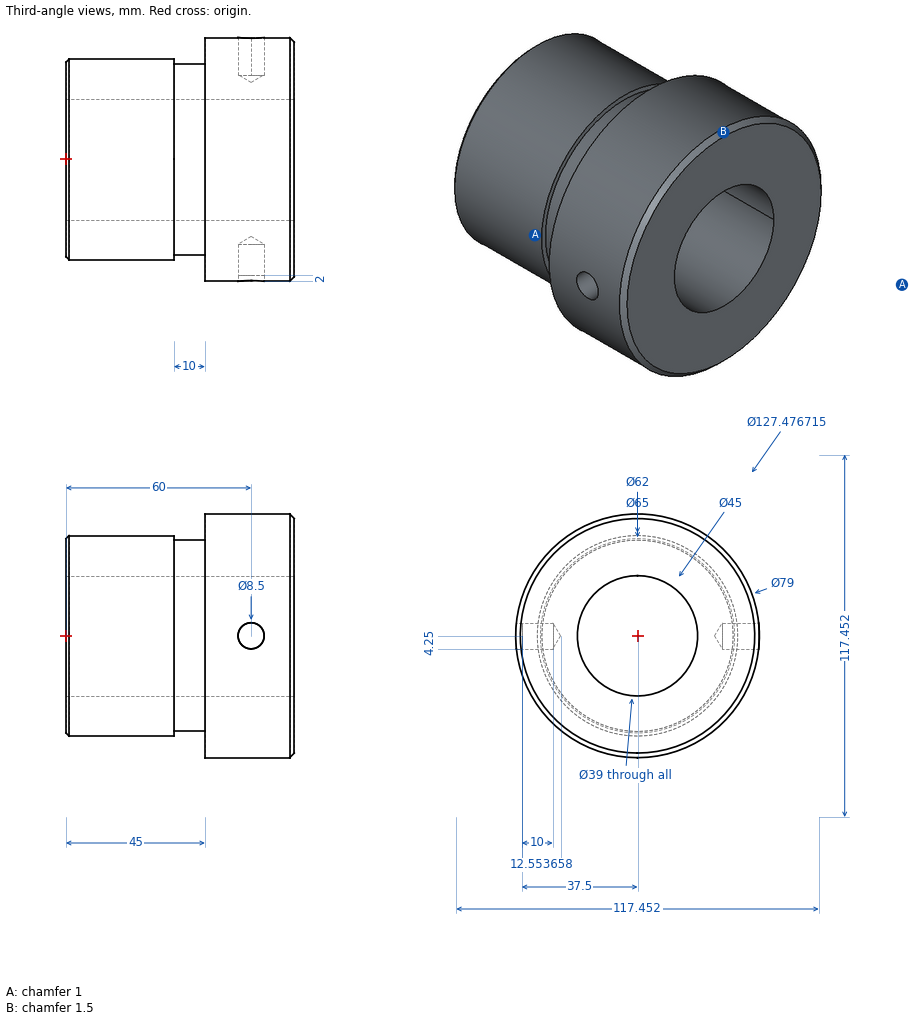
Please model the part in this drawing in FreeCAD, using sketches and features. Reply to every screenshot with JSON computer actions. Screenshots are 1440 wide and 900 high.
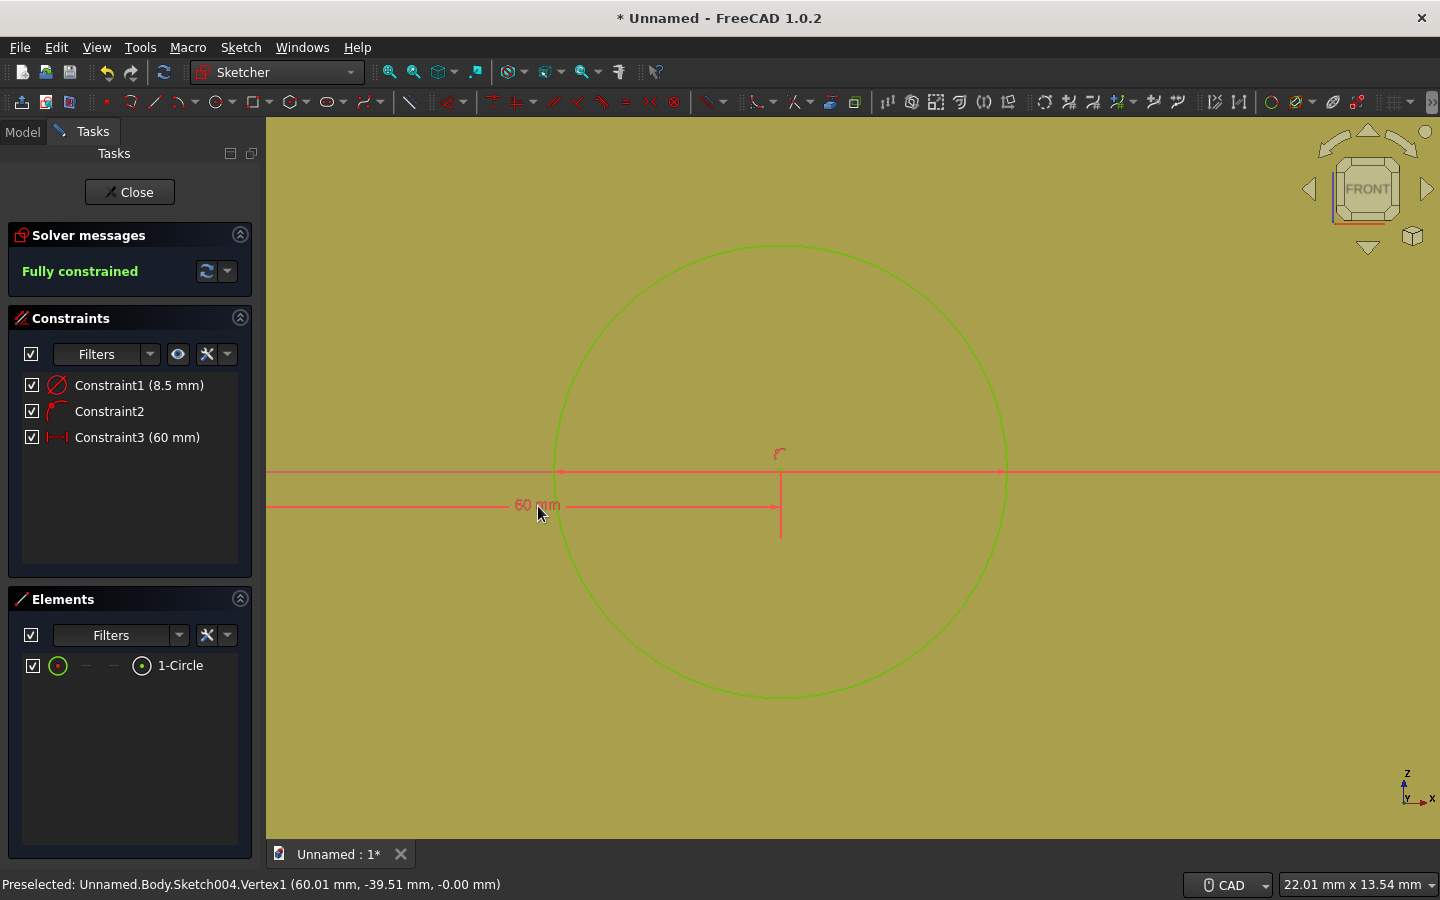
{"action": "left_click", "coordinate": [130, 192]}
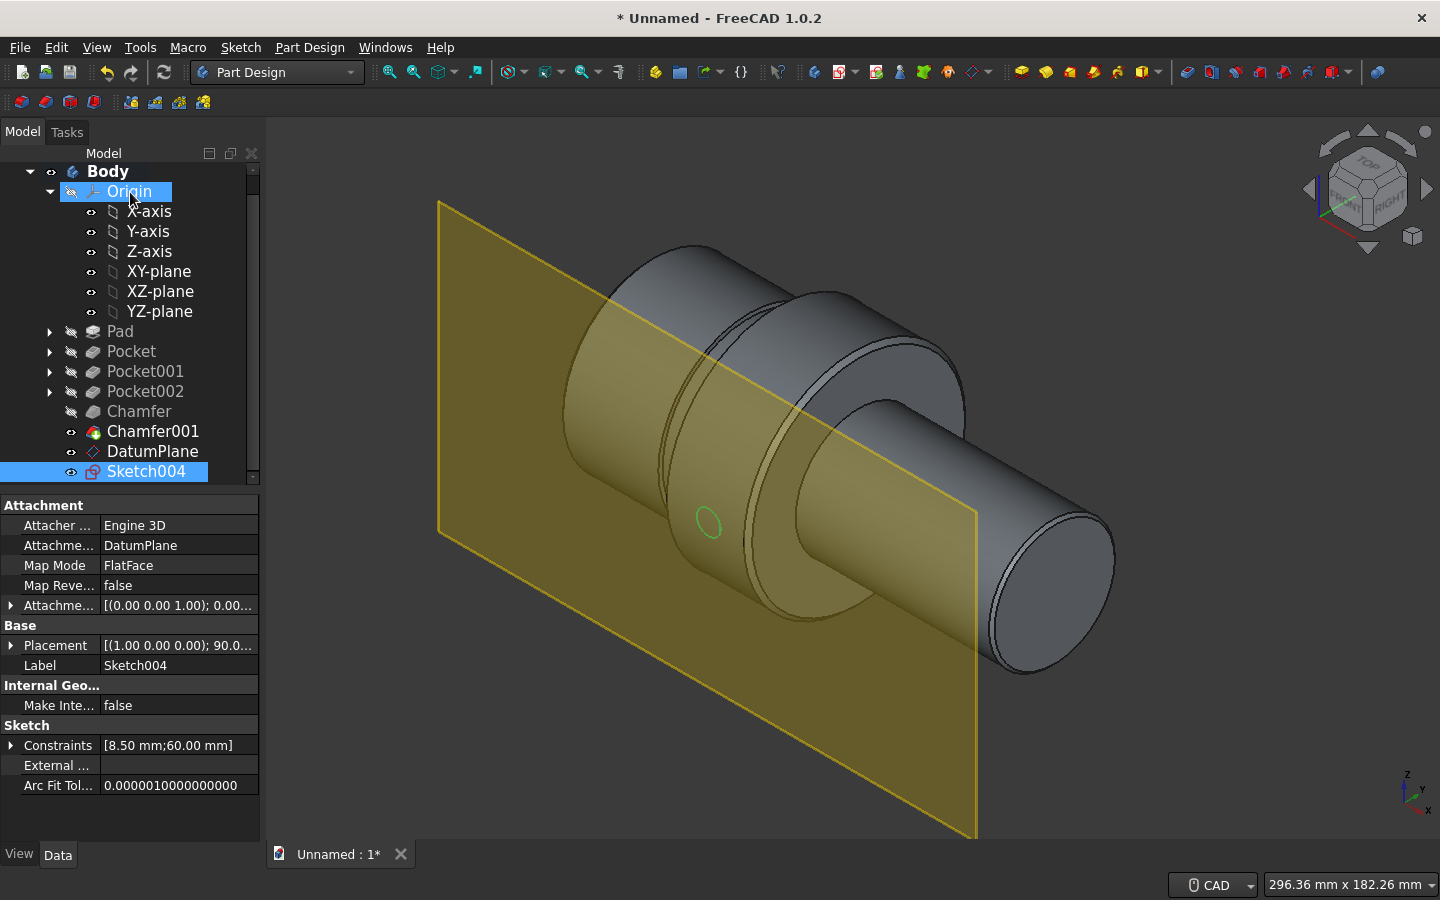
{"action": "left_click", "coordinate": [1188, 72]}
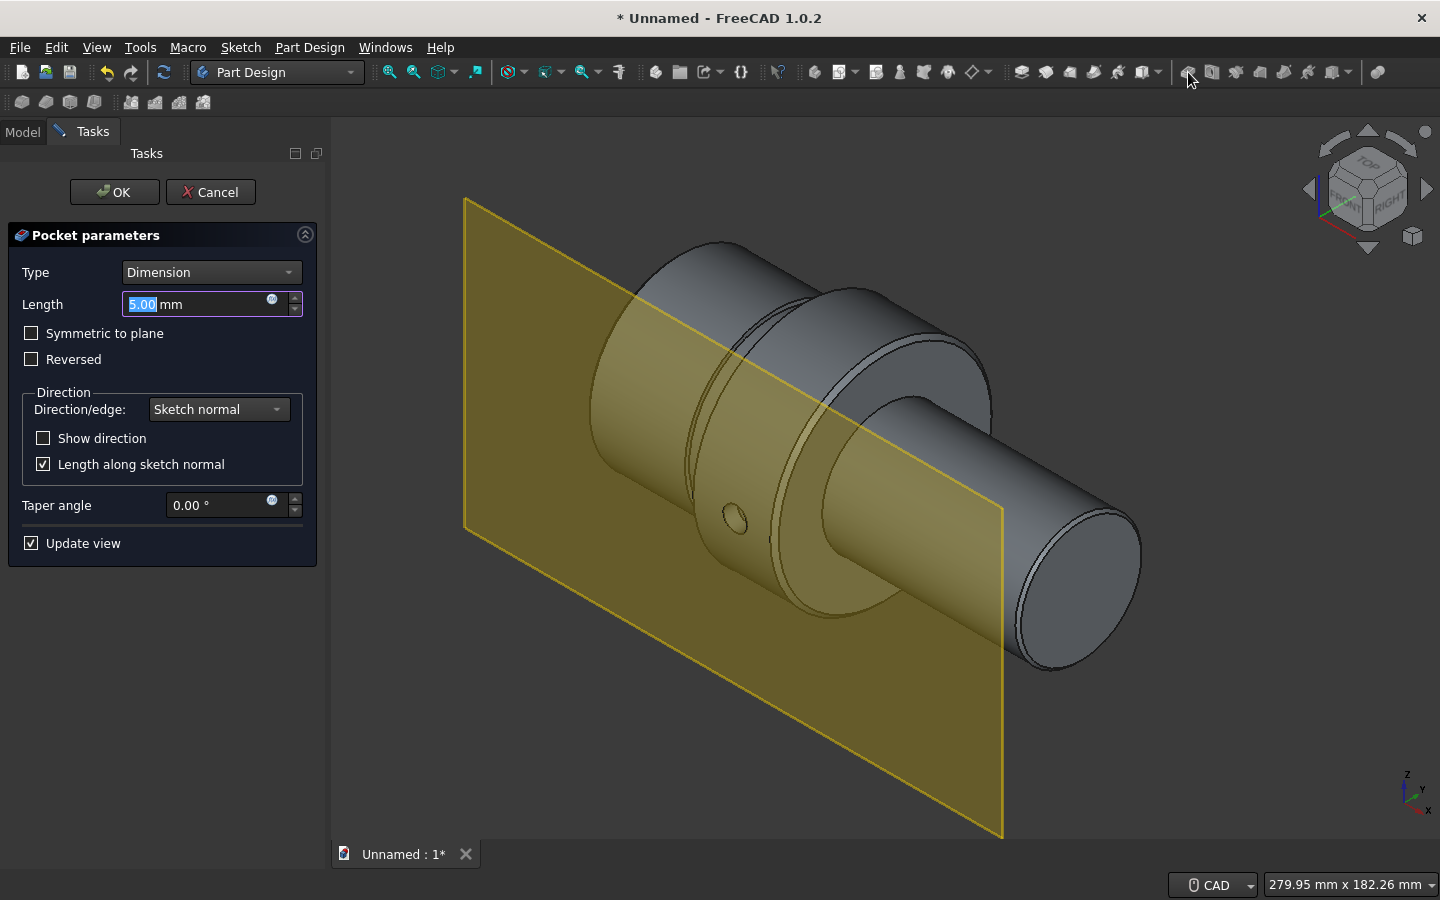
{"action": "type", "text": "2"}
{"action": "key", "text": "Tab"}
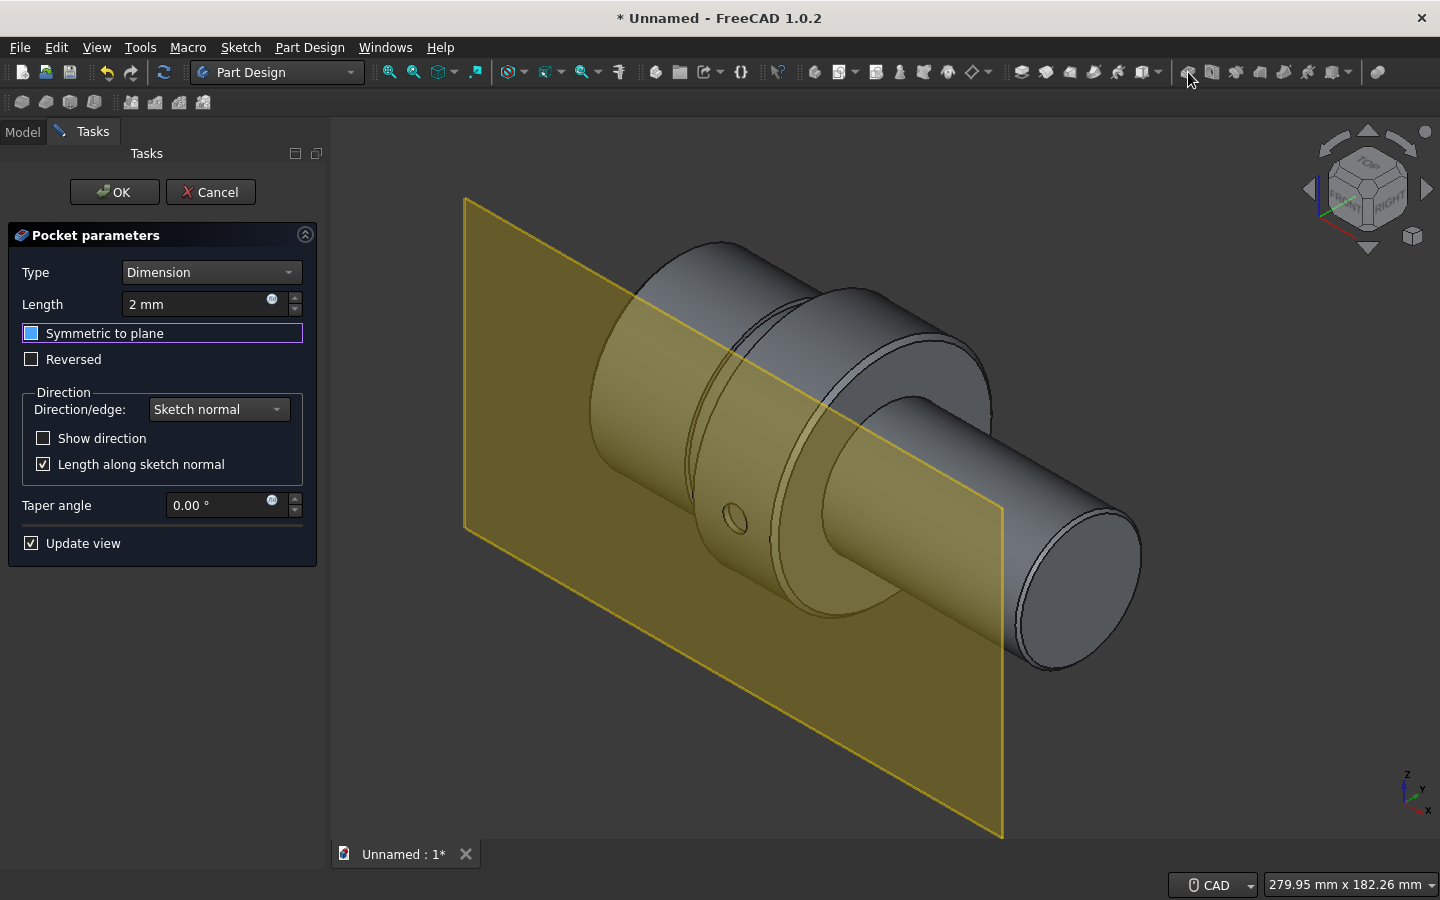
{"action": "left_click", "coordinate": [115, 192]}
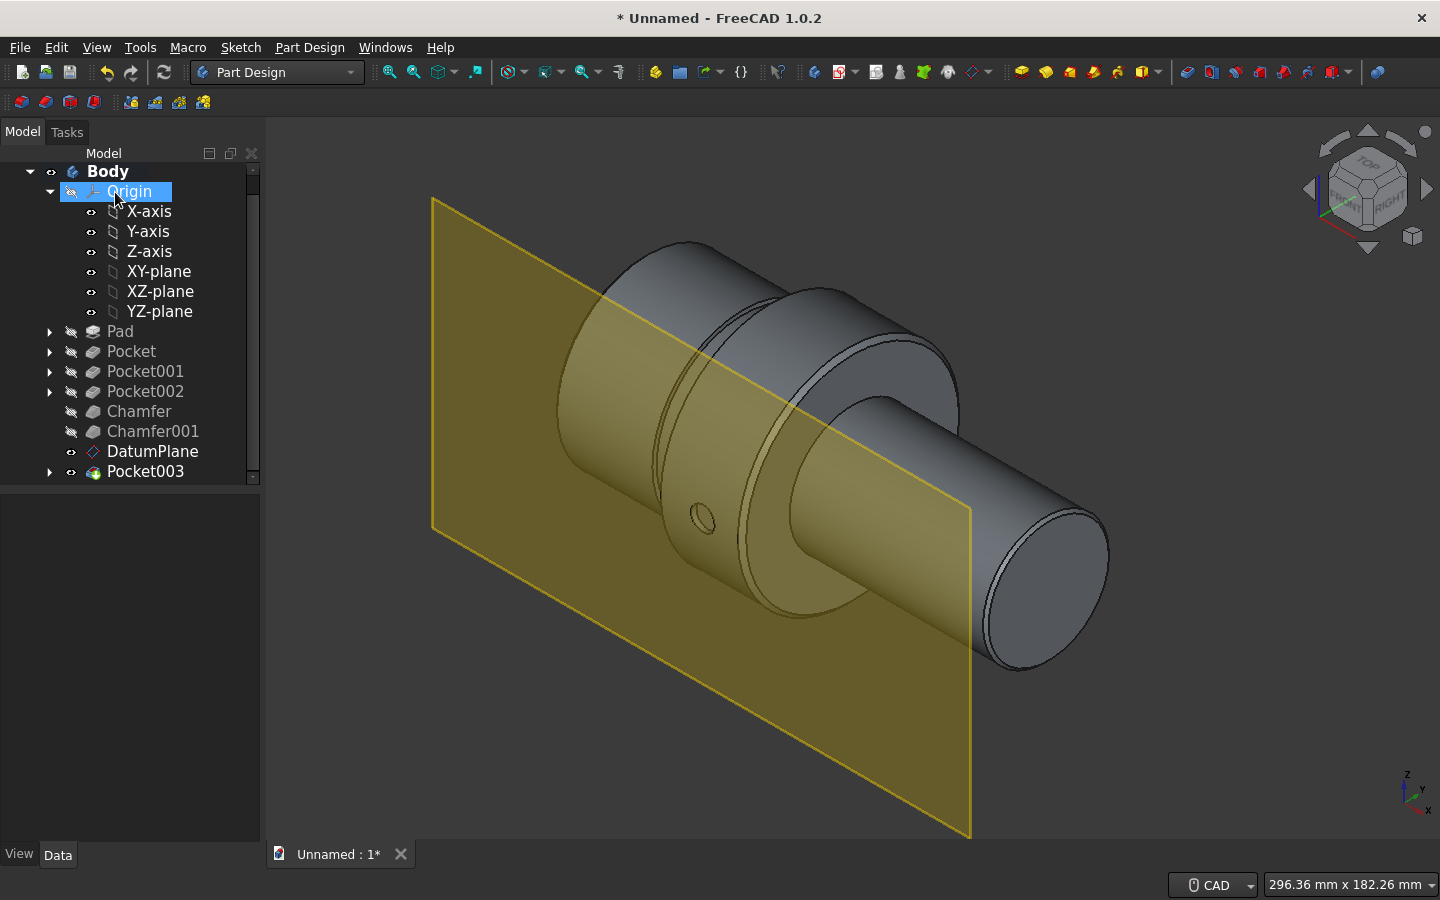
{"action": "left_click", "coordinate": [116, 452]}
{"action": "key", "text": "space"}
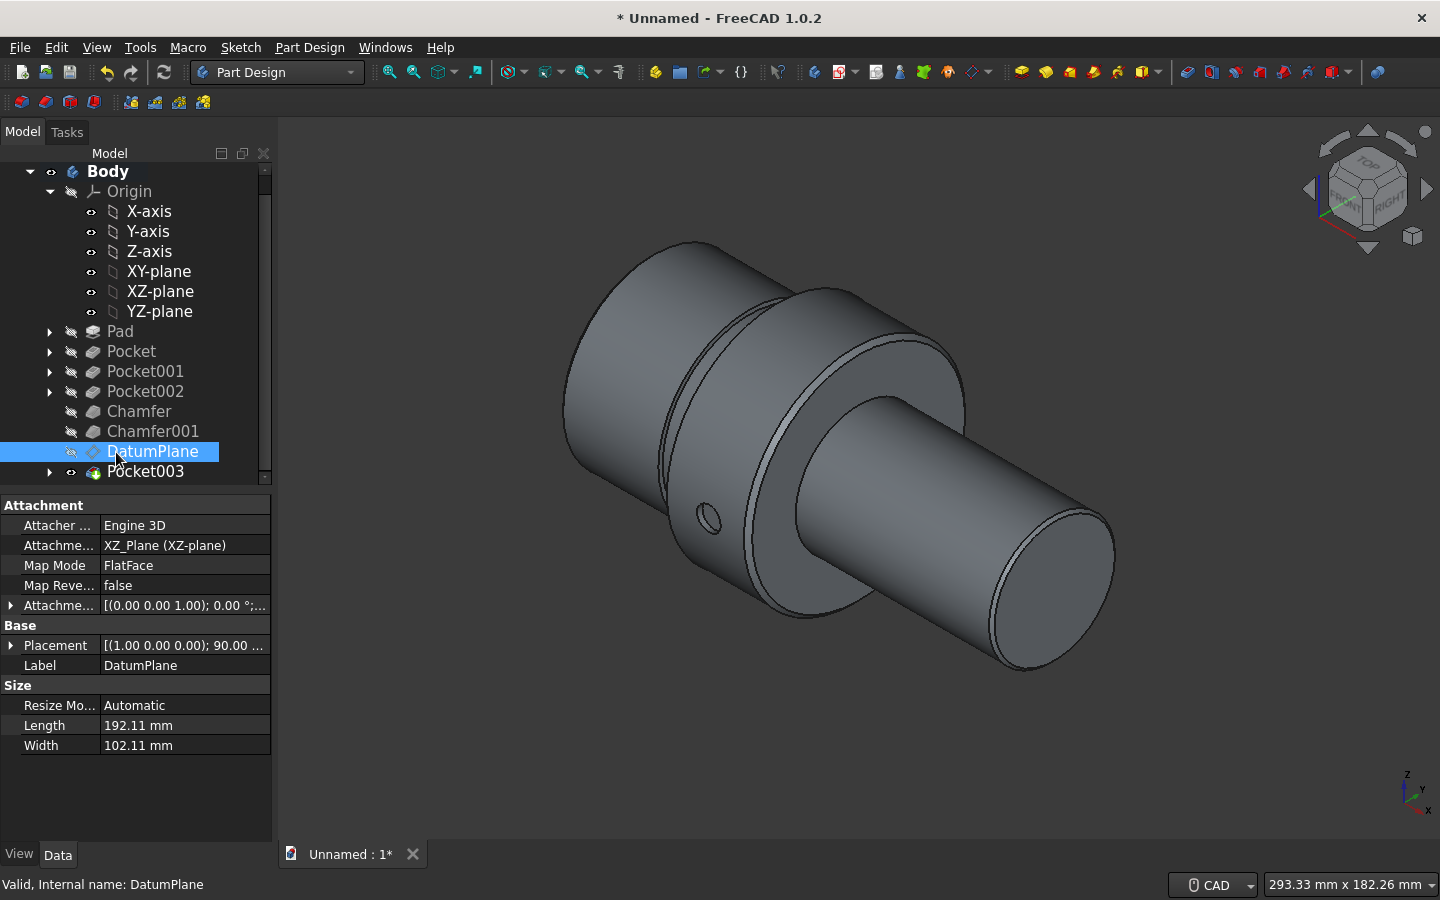
{"action": "left_click", "coordinate": [136, 312]}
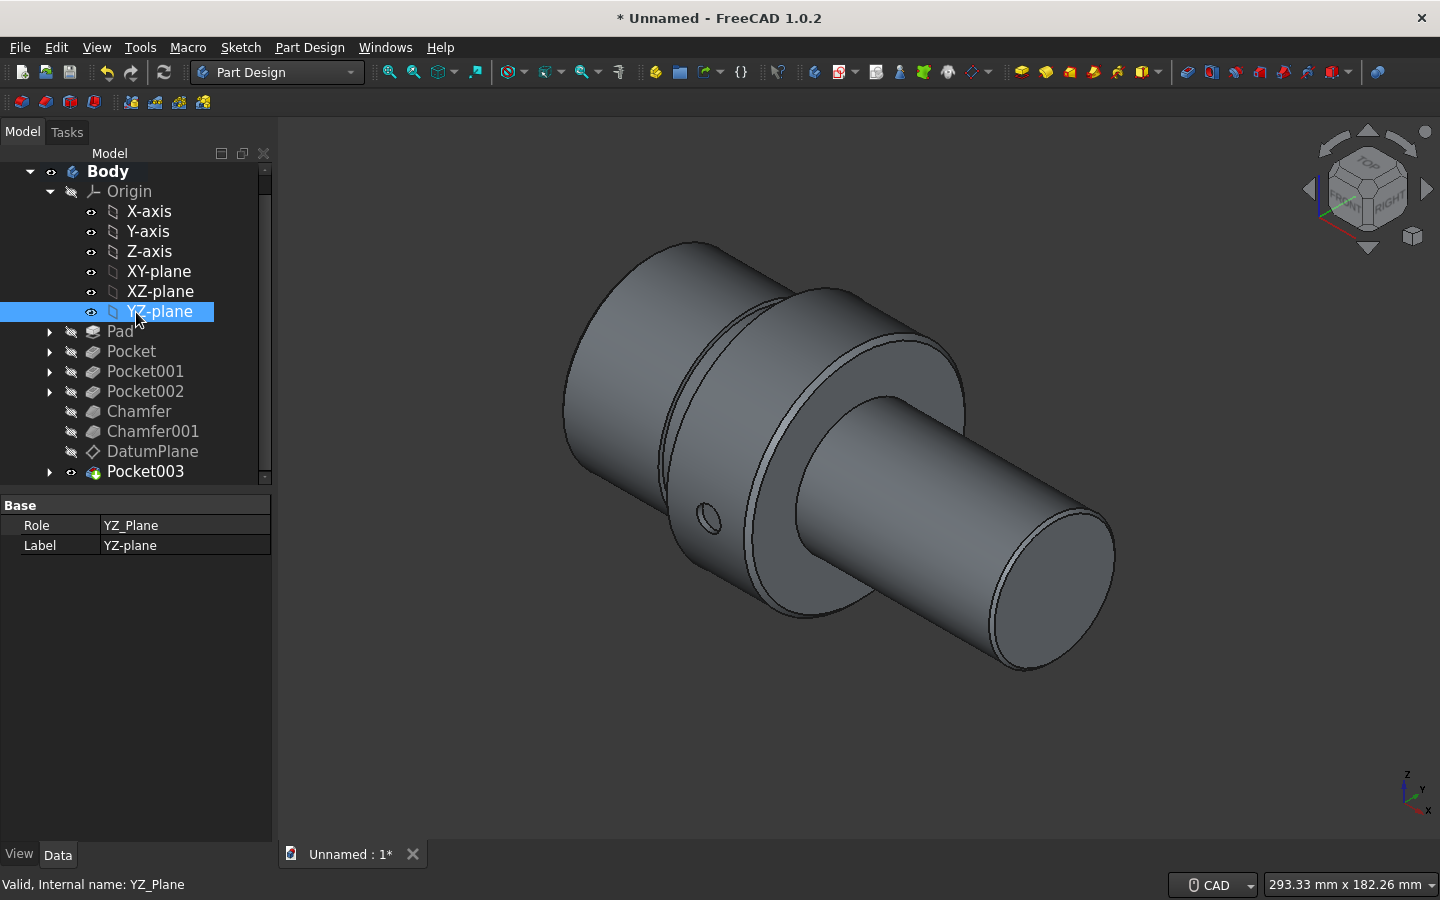
{"action": "left_click", "coordinate": [972, 72]}